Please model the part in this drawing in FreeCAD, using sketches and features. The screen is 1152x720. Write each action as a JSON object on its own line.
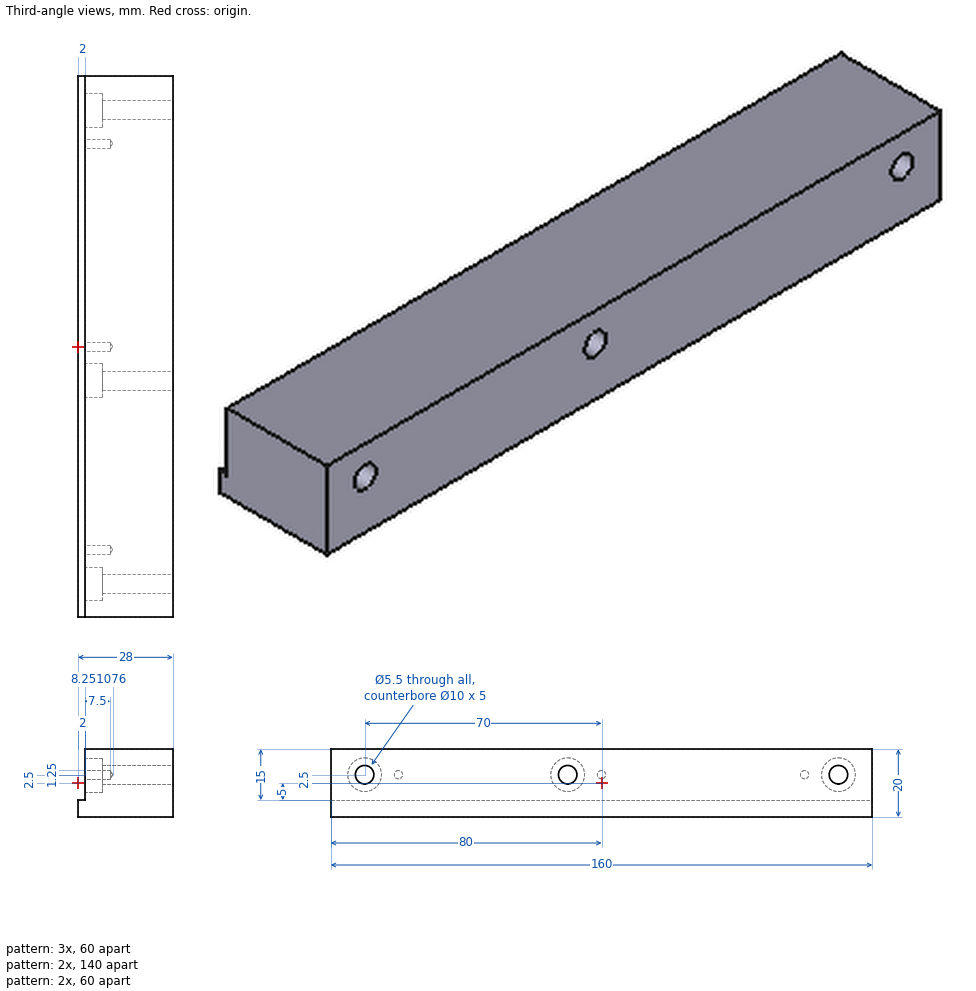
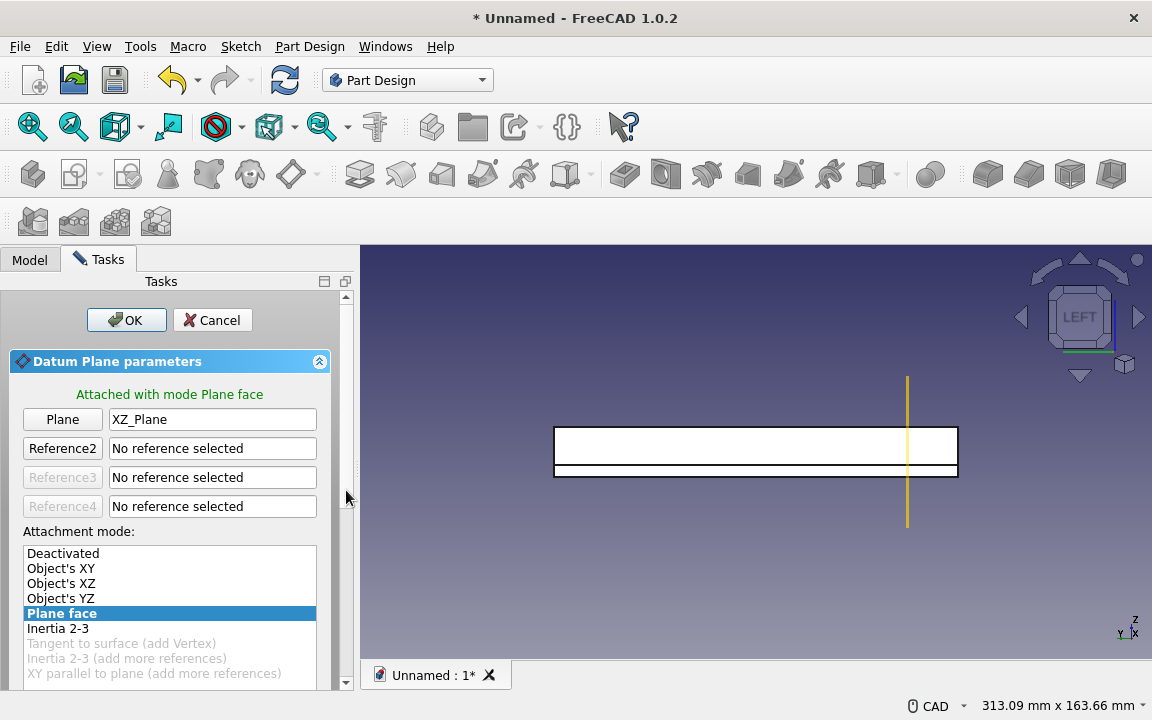
{"action": "left_click", "coordinate": [127, 320]}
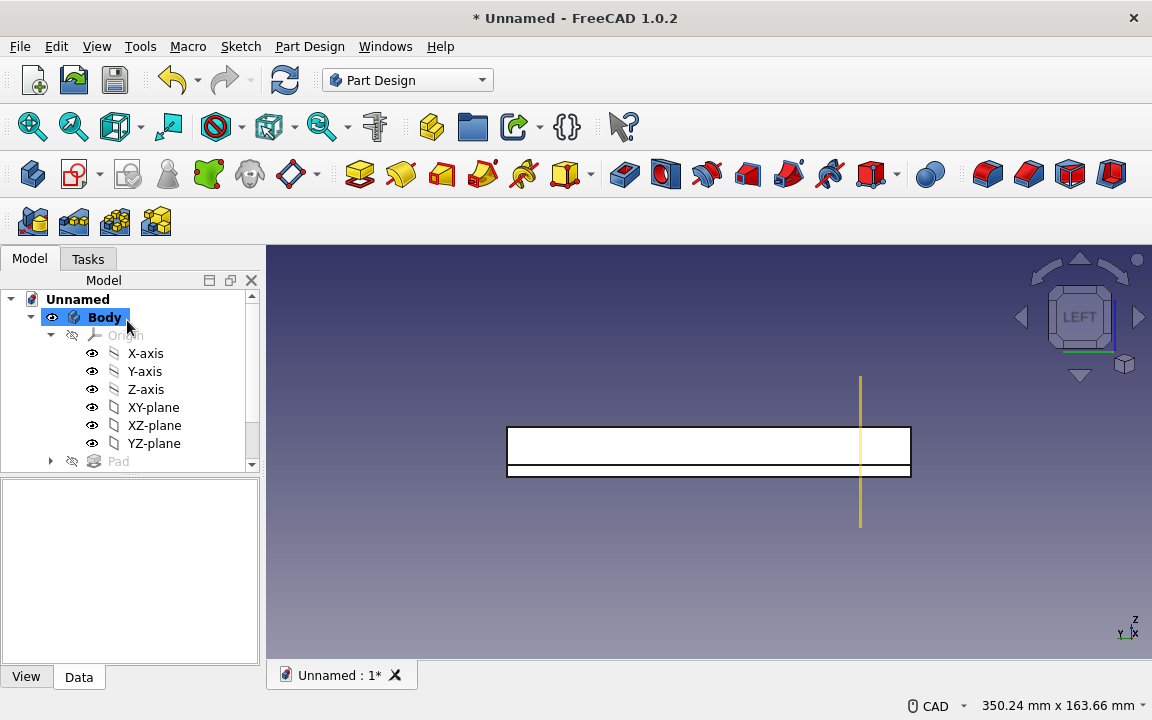
{"action": "scroll", "coordinate": [101, 385], "scroll_direction": "down", "scroll_amount": 3}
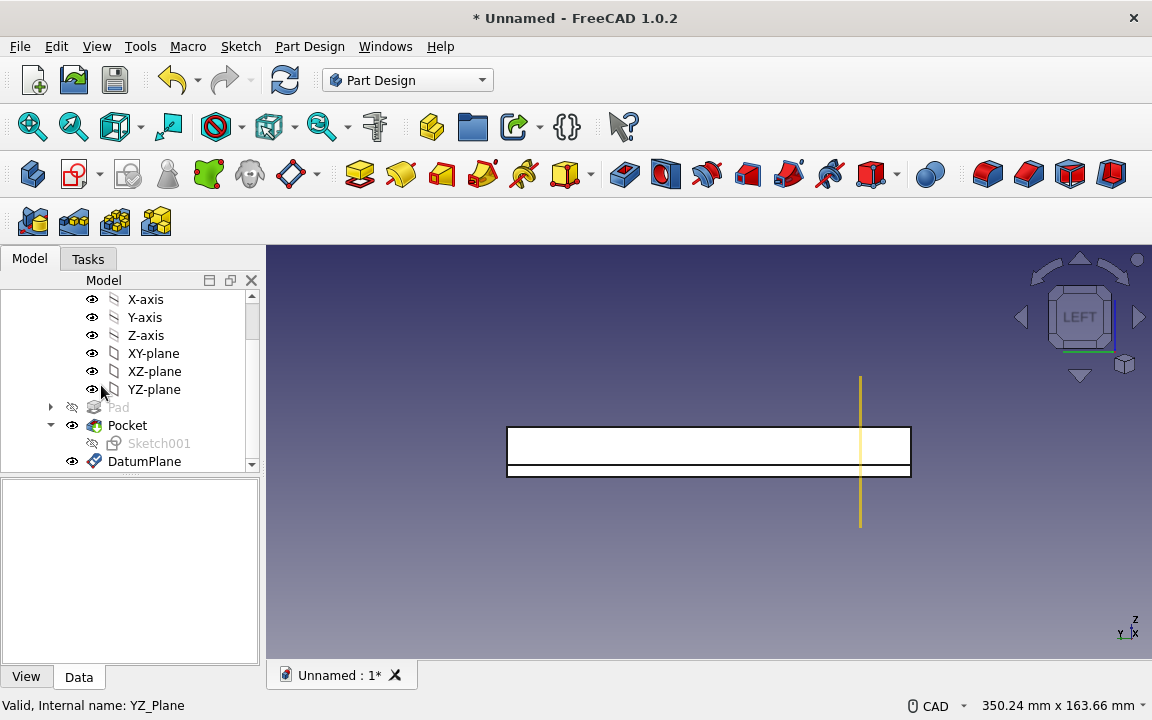
{"action": "left_click", "coordinate": [117, 461]}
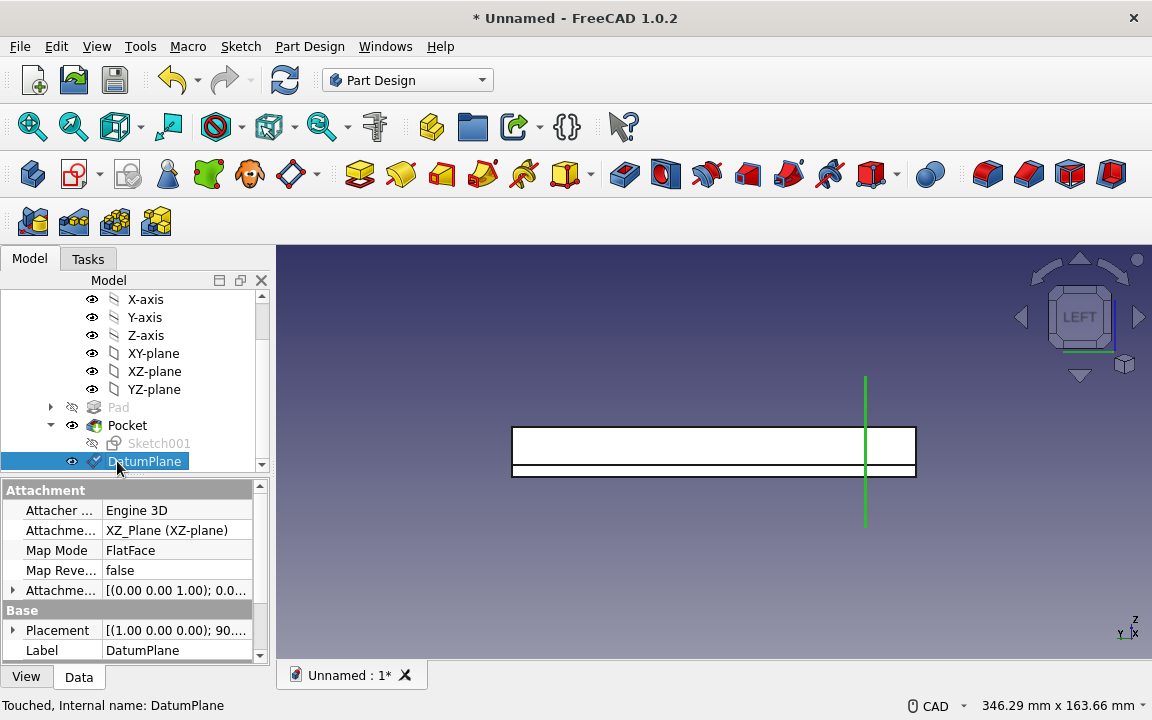
{"action": "left_click", "coordinate": [74, 174]}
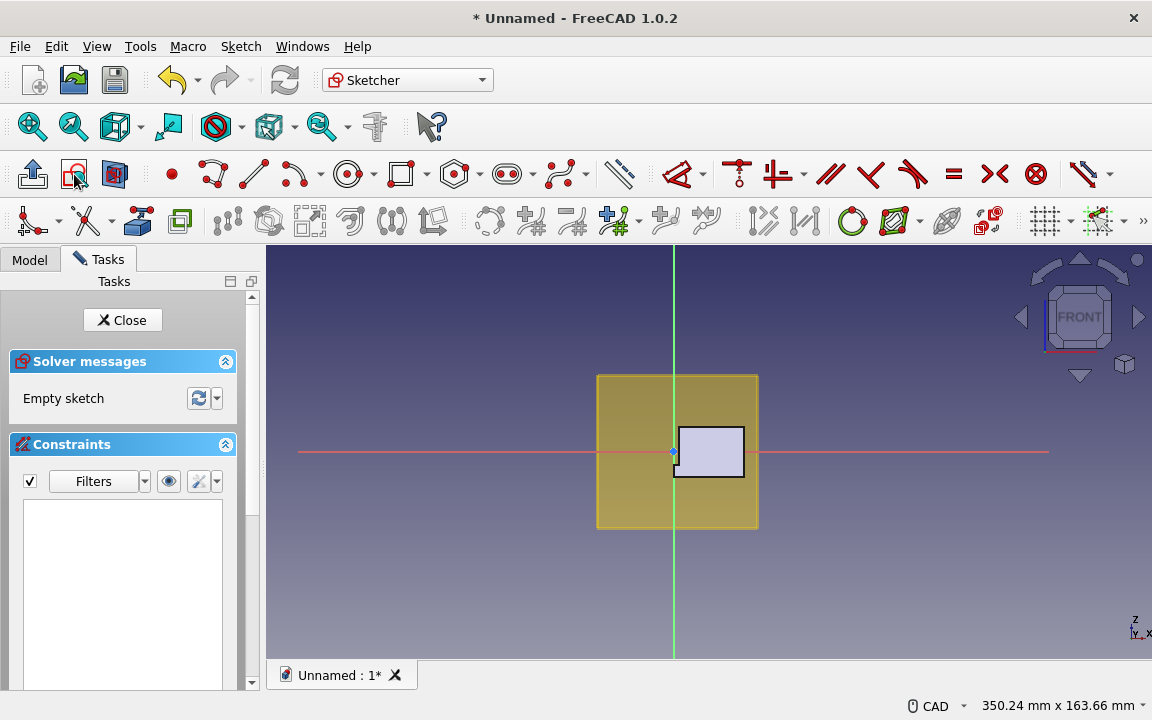
{"action": "left_click", "coordinate": [115, 174]}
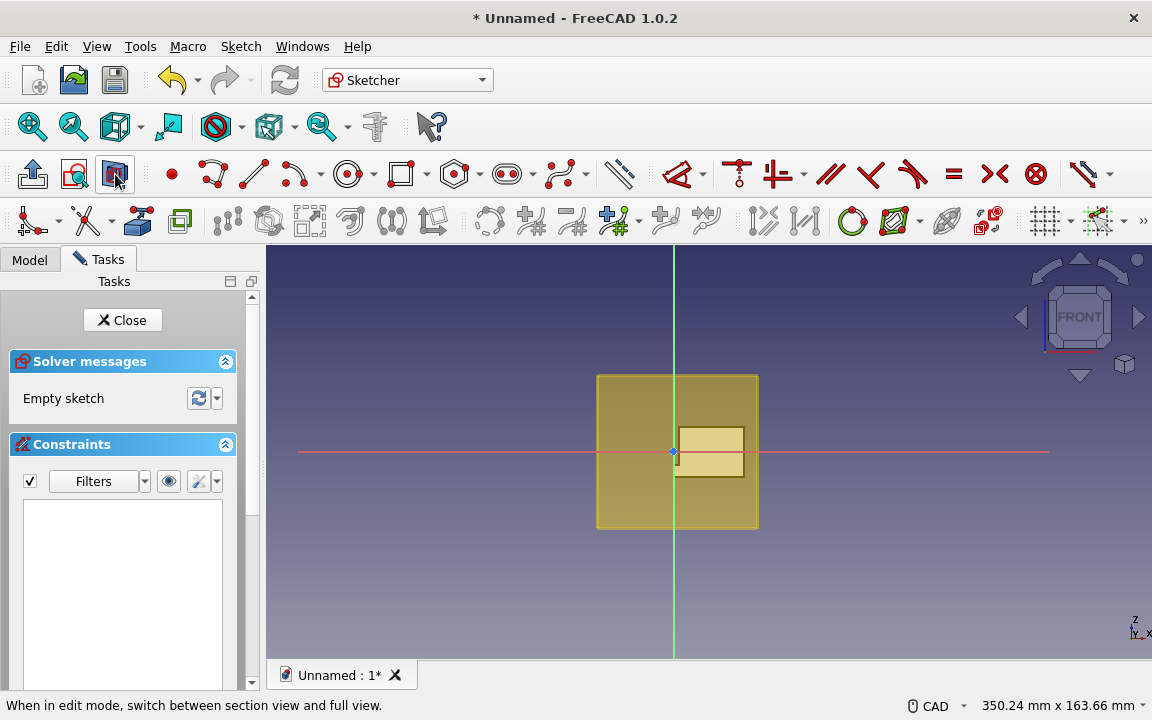
{"action": "scroll", "coordinate": [695, 447], "scroll_direction": "up", "scroll_amount": 13}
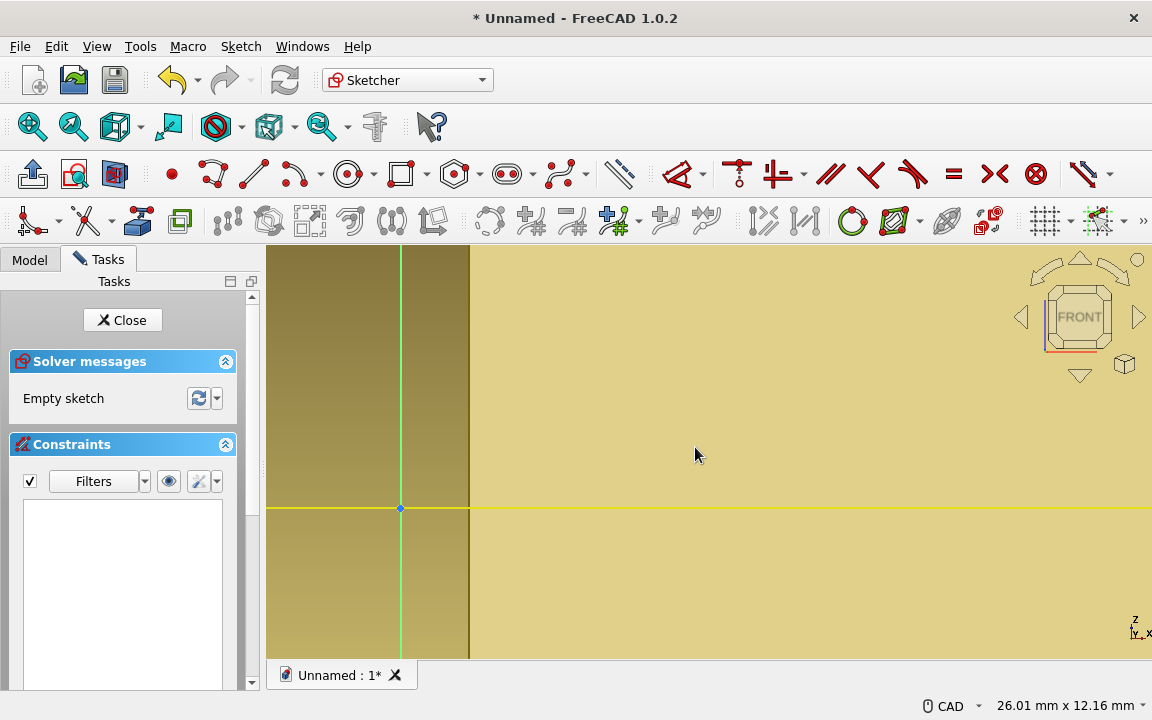
{"action": "key", "text": "g m"}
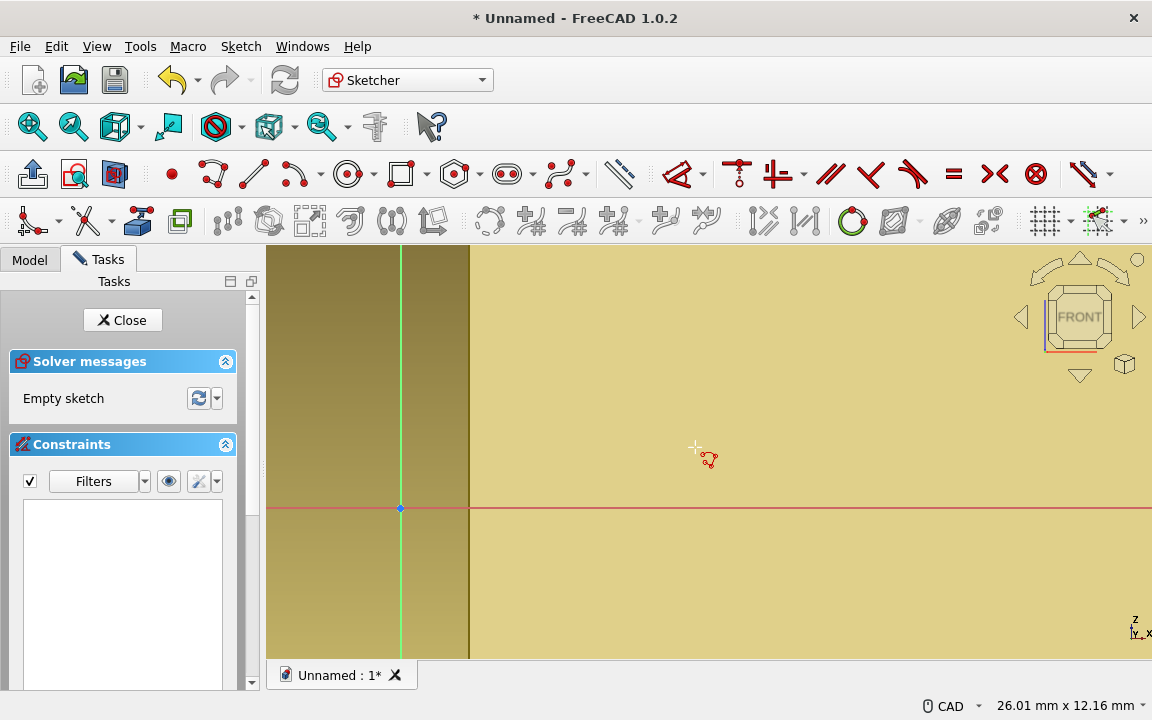
{"action": "left_click", "coordinate": [469, 423]}
{"action": "left_click", "coordinate": [469, 381]}
{"action": "left_click", "coordinate": [724, 381]}
{"action": "left_click", "coordinate": [750, 423]}
{"action": "left_click", "coordinate": [469, 424]}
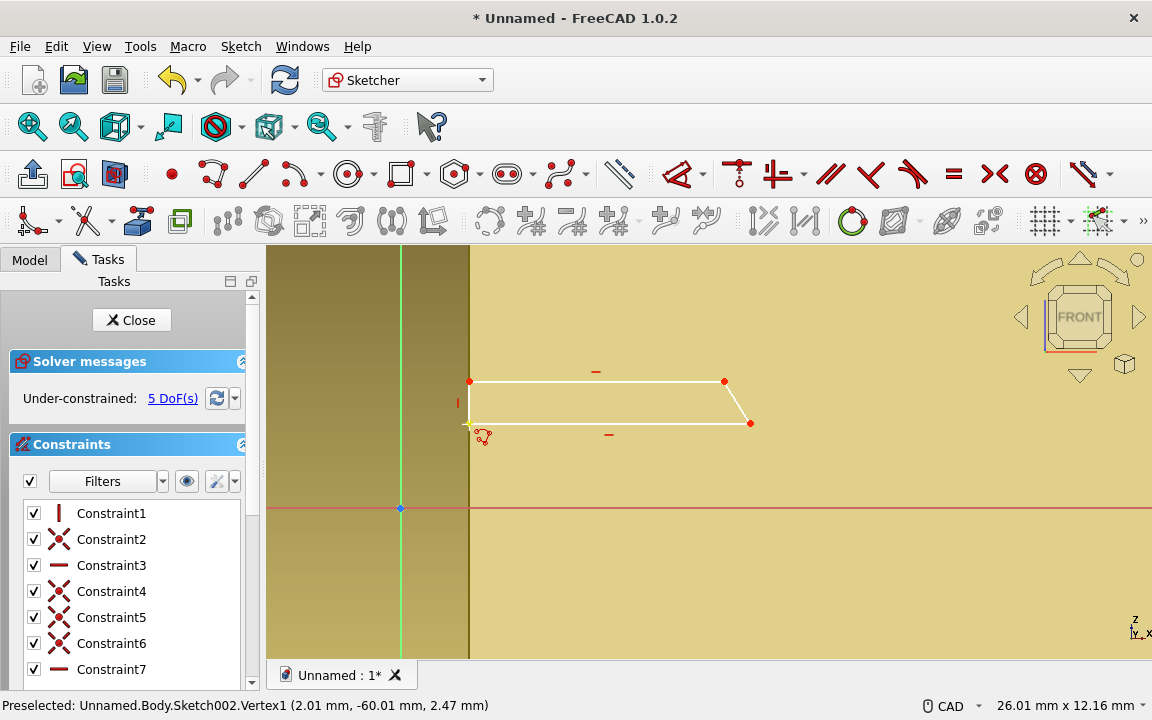
{"action": "key", "text": "g l"}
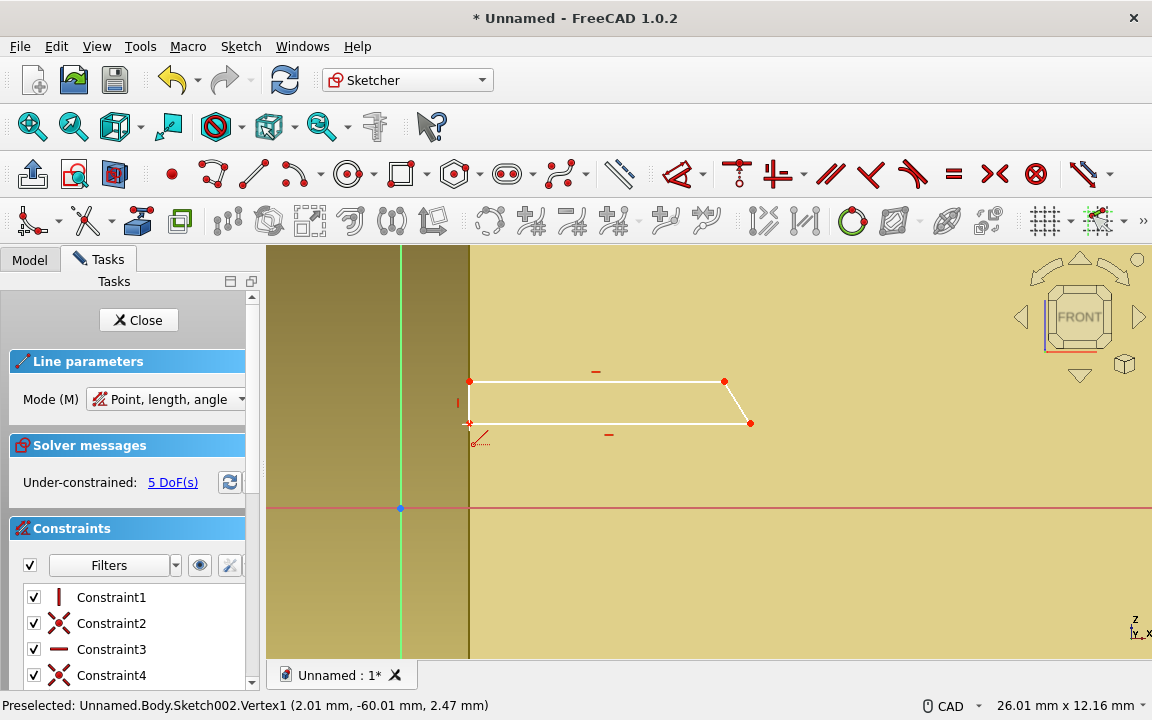
{"action": "left_click", "coordinate": [778, 423]}
{"action": "left_click", "coordinate": [862, 423]}
{"action": "key", "text": "Escape"}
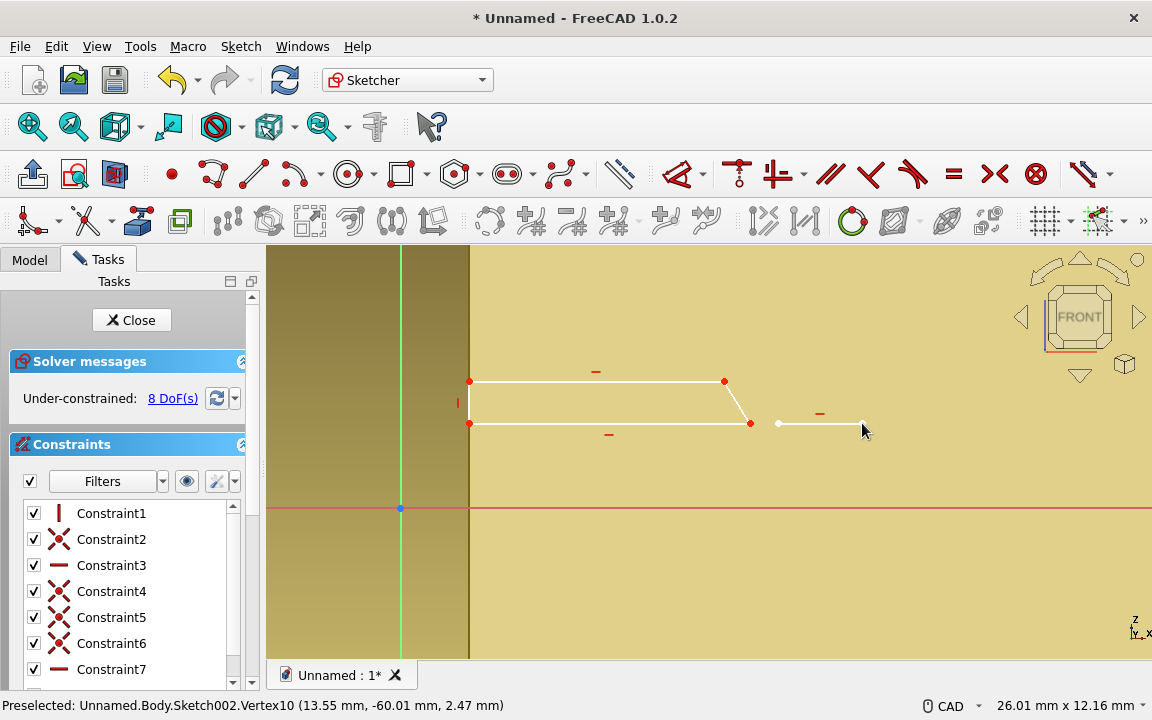
{"action": "left_click", "coordinate": [803, 424]}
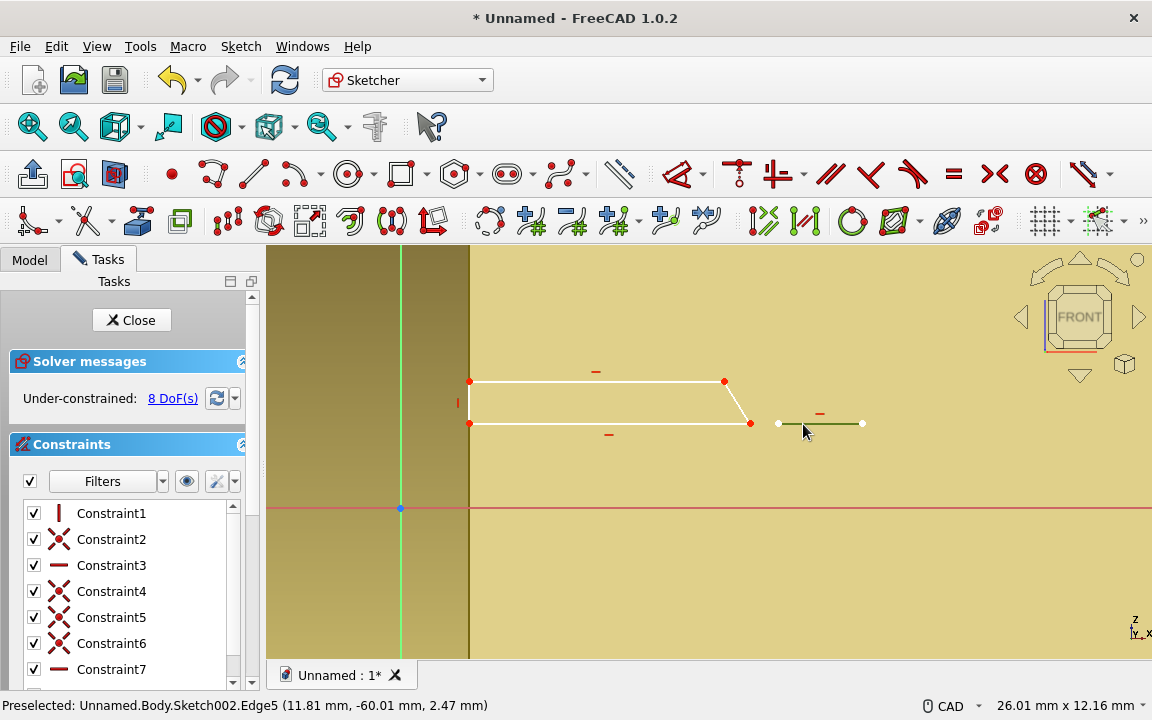
{"action": "left_click", "coordinate": [620, 174]}